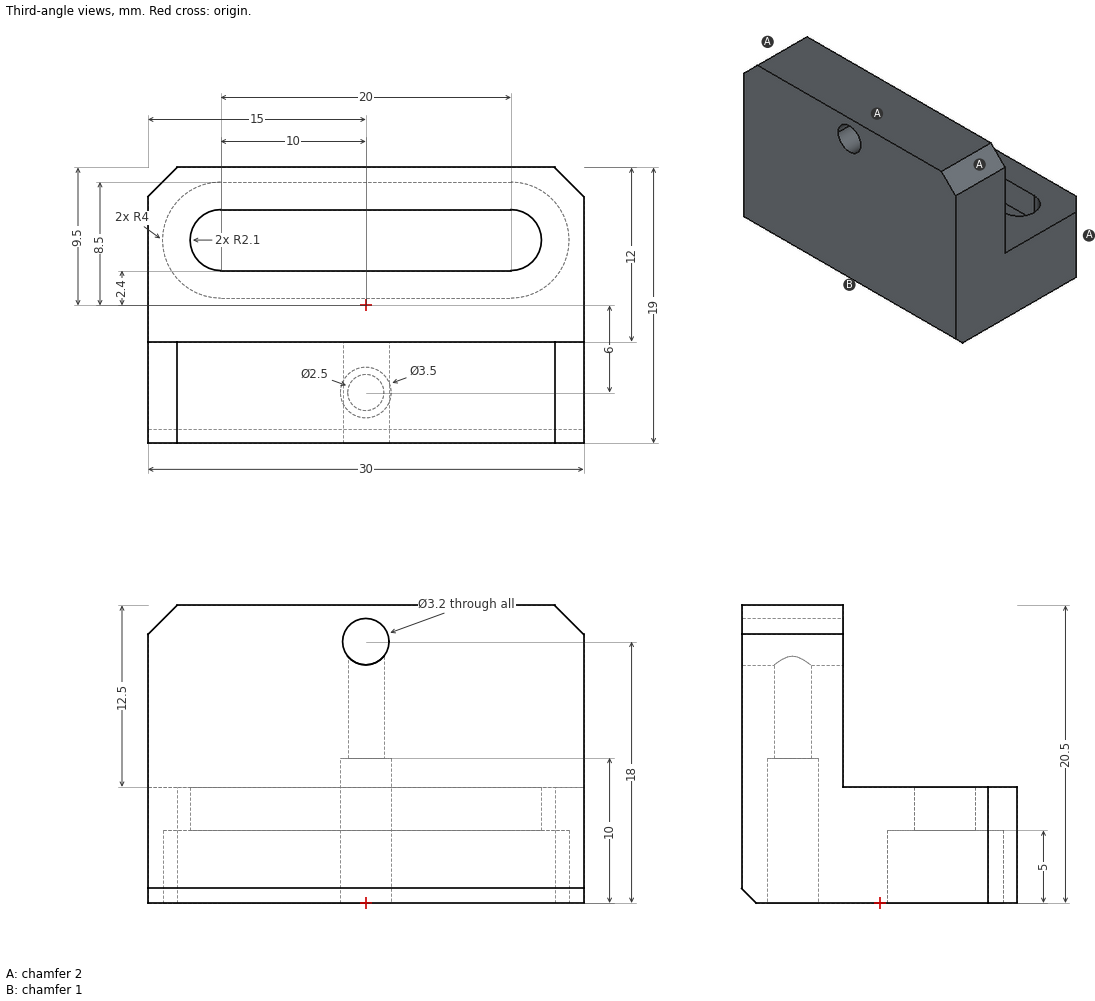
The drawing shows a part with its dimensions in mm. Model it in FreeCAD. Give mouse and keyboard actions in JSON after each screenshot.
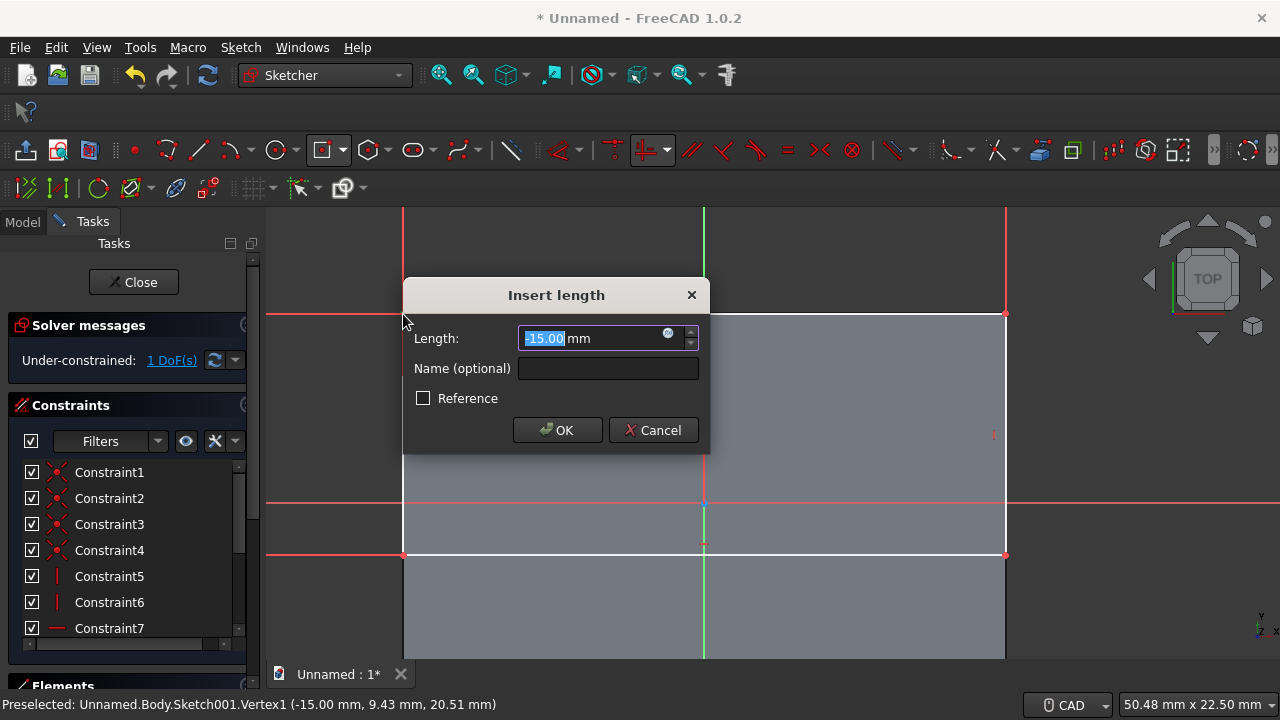
{"action": "type", "text": "-15"}
{"action": "key", "text": "Return"}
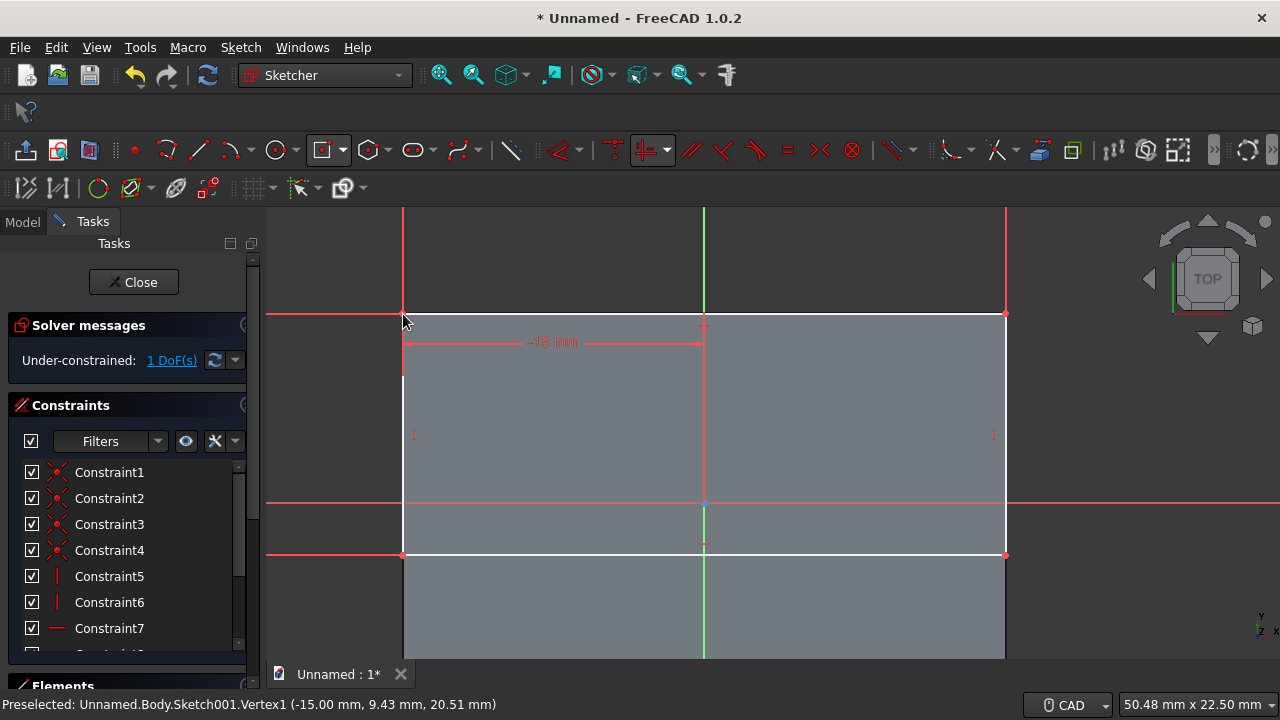
{"action": "left_click", "coordinate": [403, 314]}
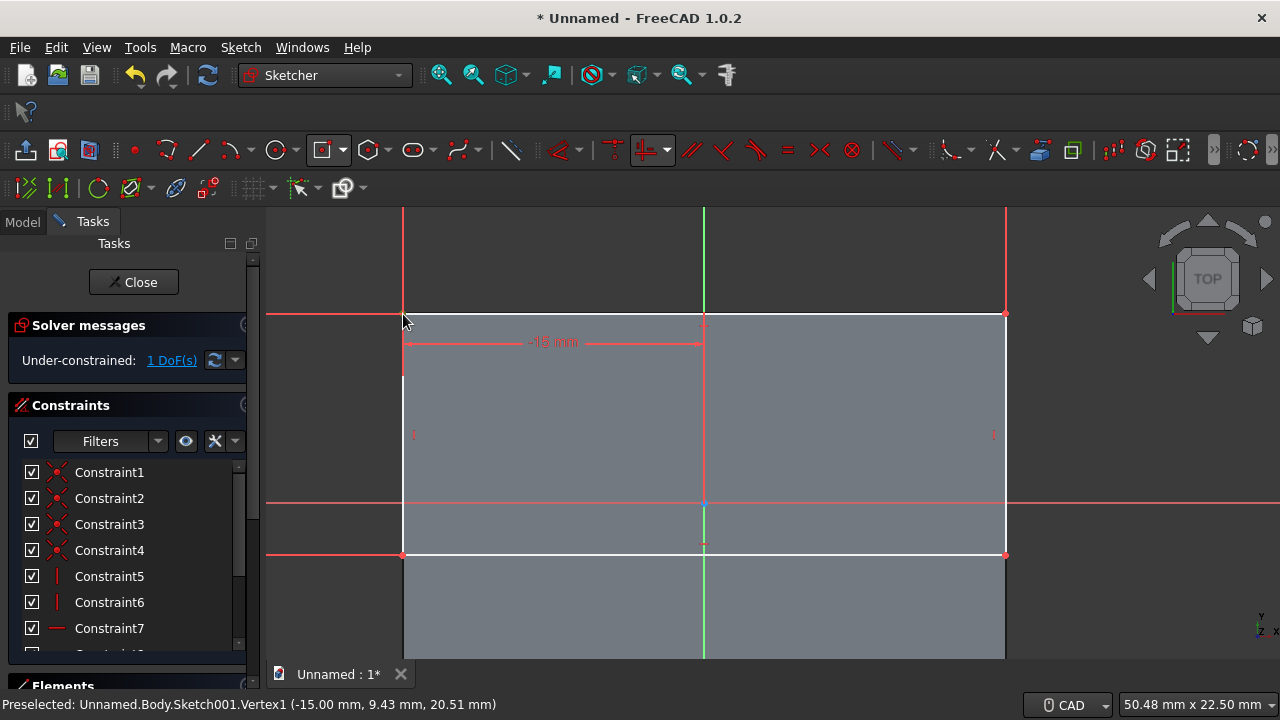
{"action": "left_click", "coordinate": [582, 150]}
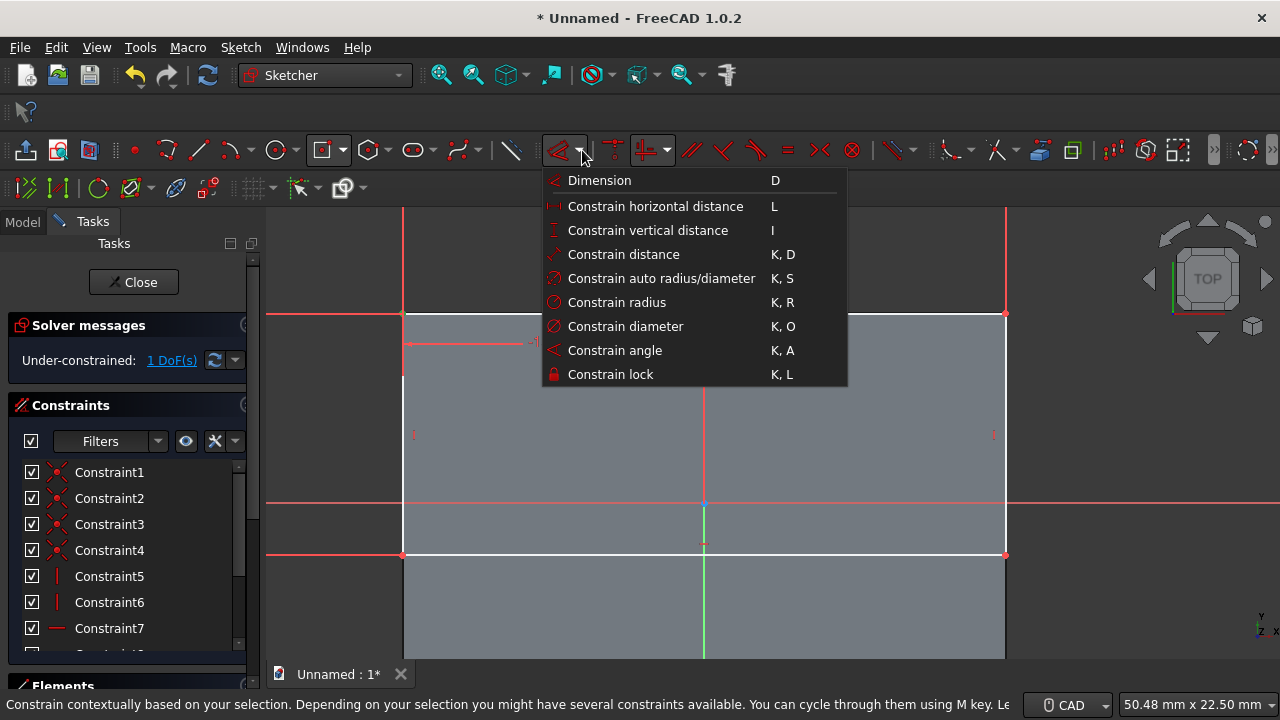
{"action": "left_click", "coordinate": [695, 230]}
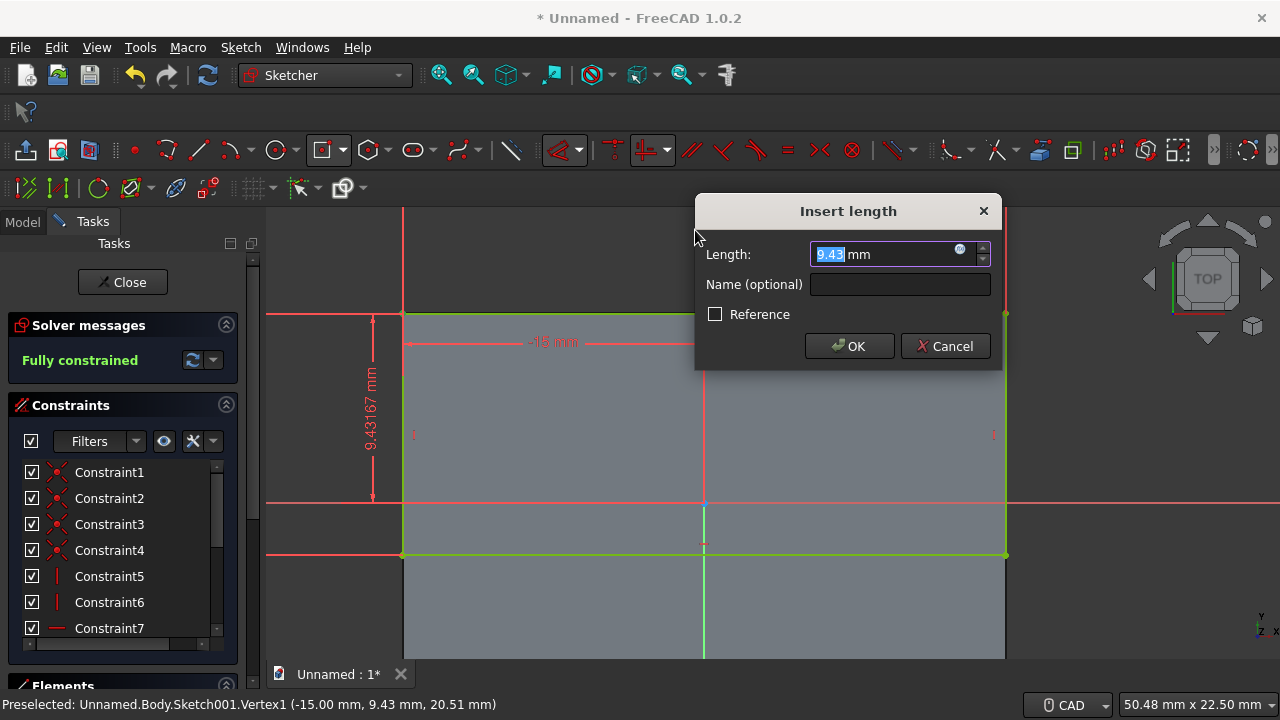
{"action": "type", "text": "9.5"}
{"action": "key", "text": "Return"}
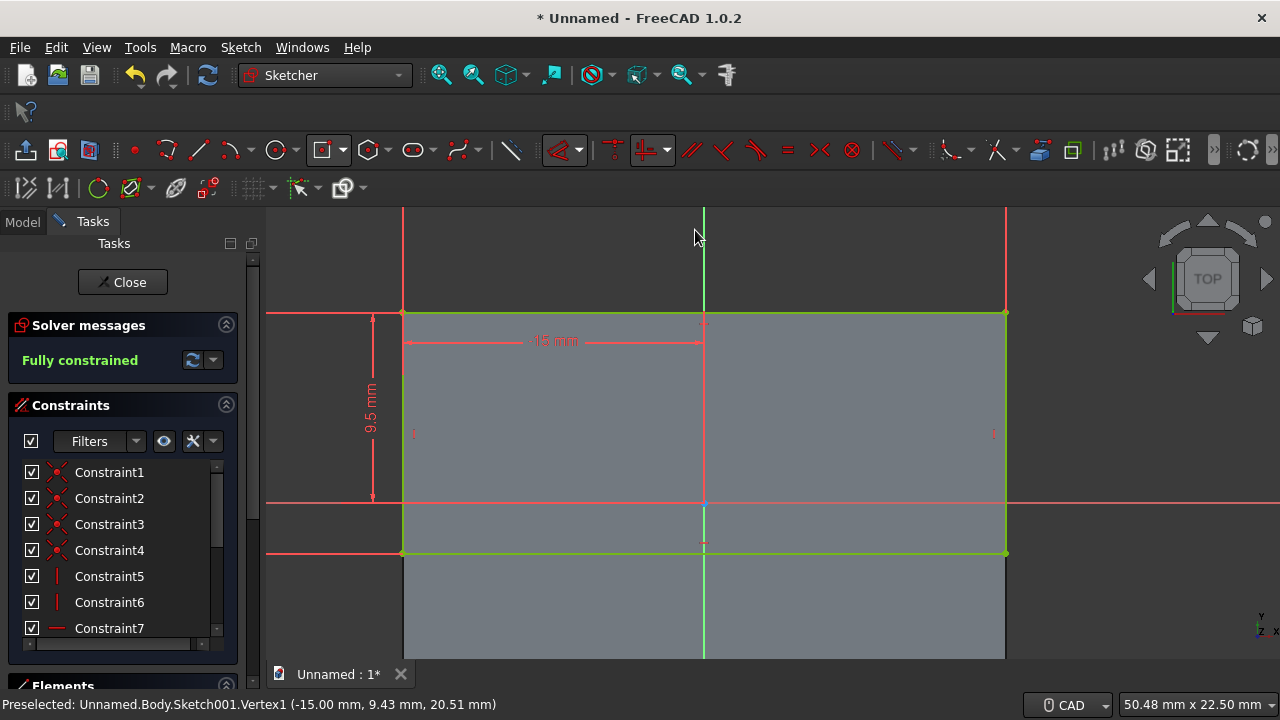
{"action": "left_click", "coordinate": [123, 282]}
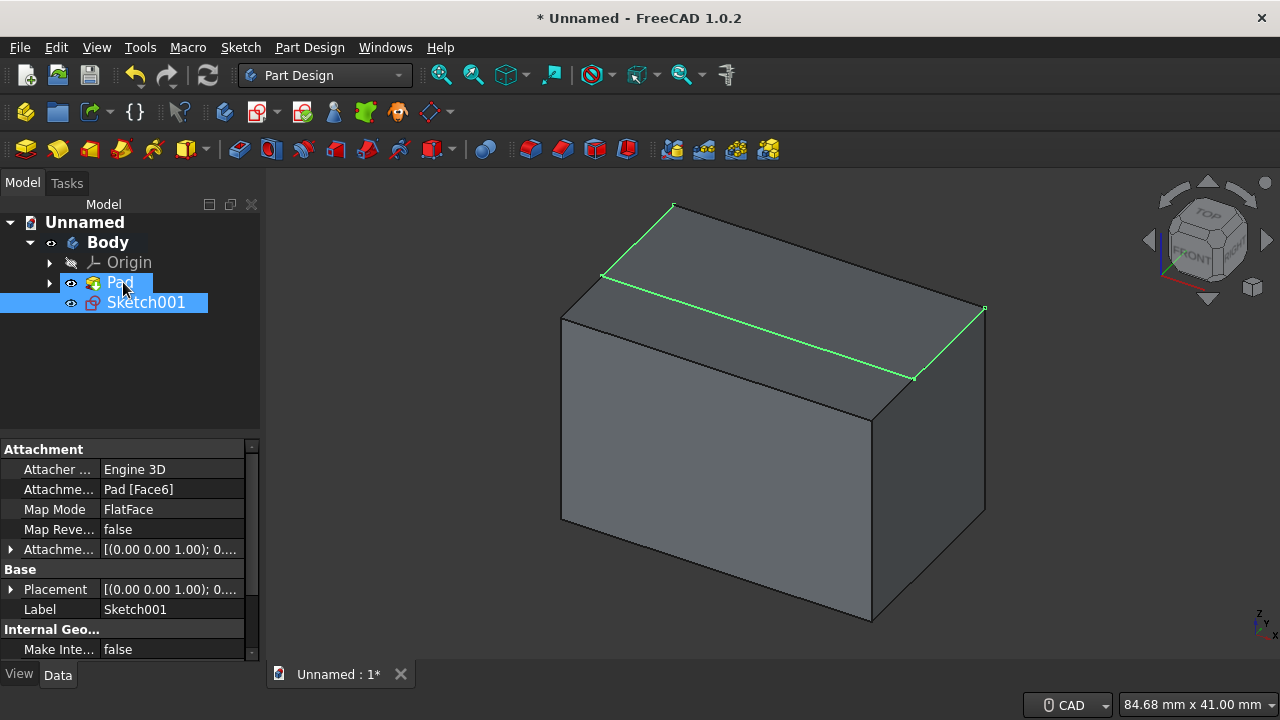
{"action": "left_click", "coordinate": [240, 150]}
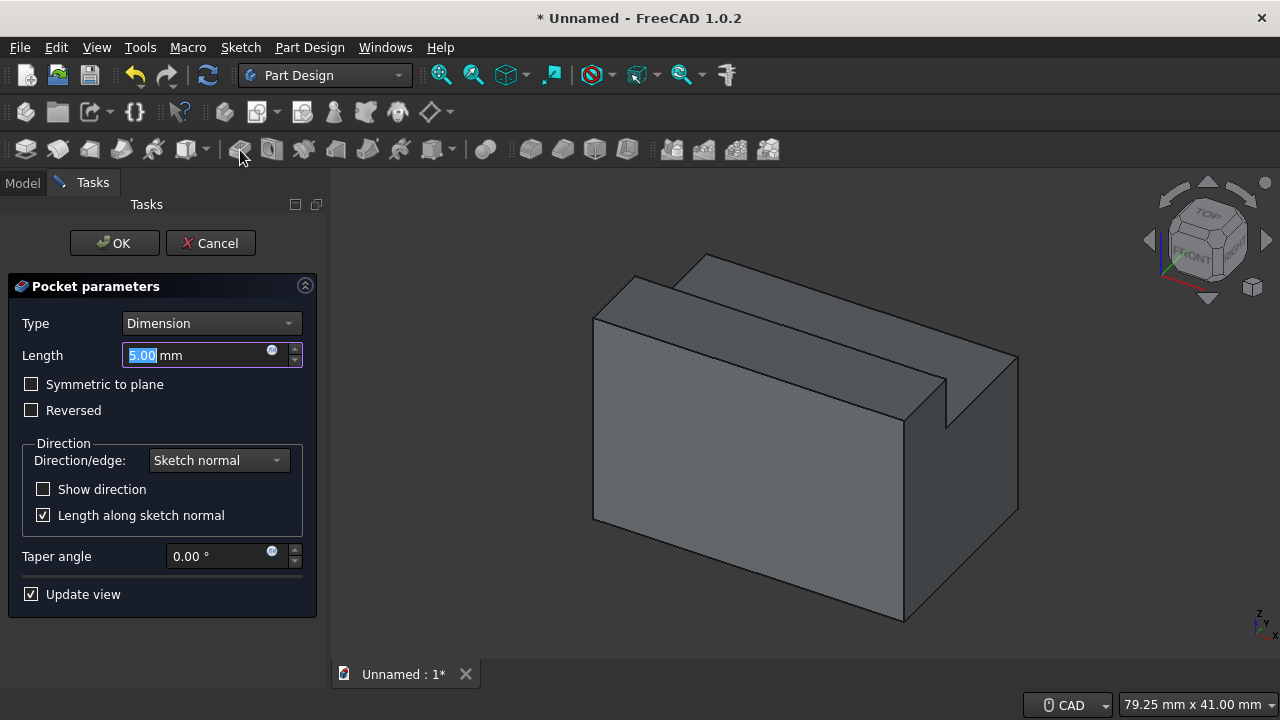
{"action": "type", "text": "12.5"}
{"action": "key", "text": "Tab"}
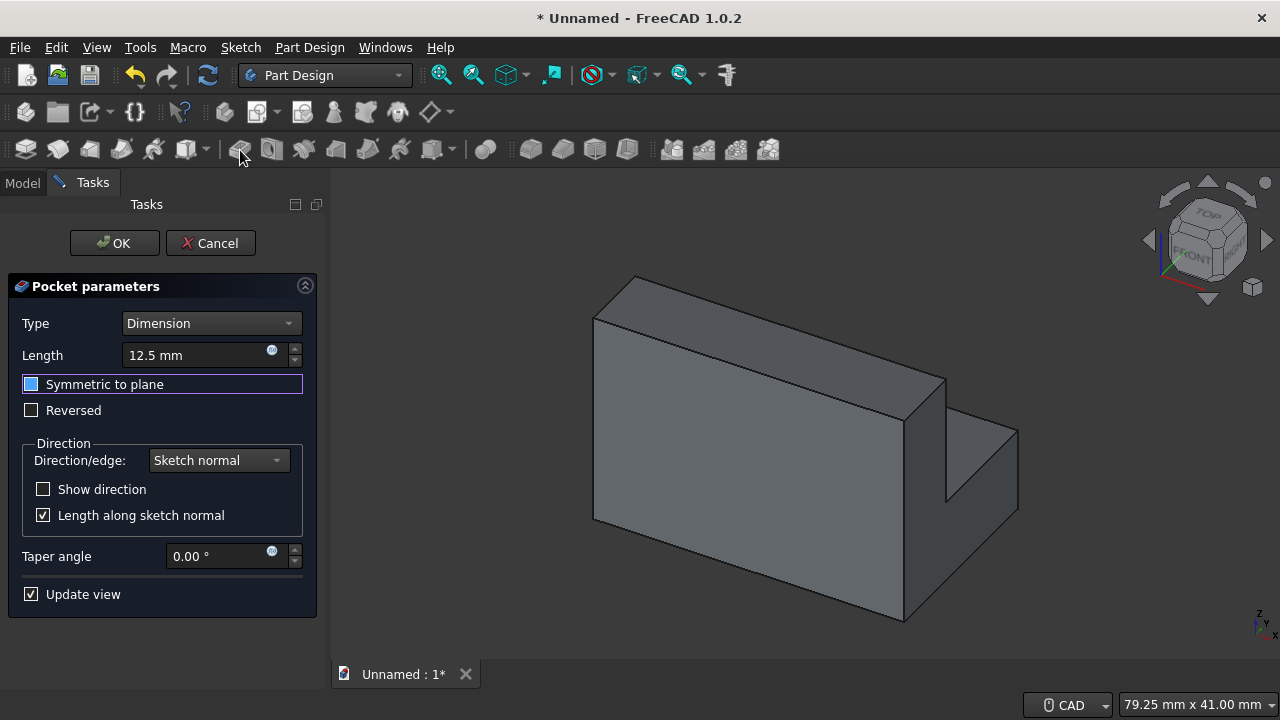
{"action": "left_click", "coordinate": [115, 243]}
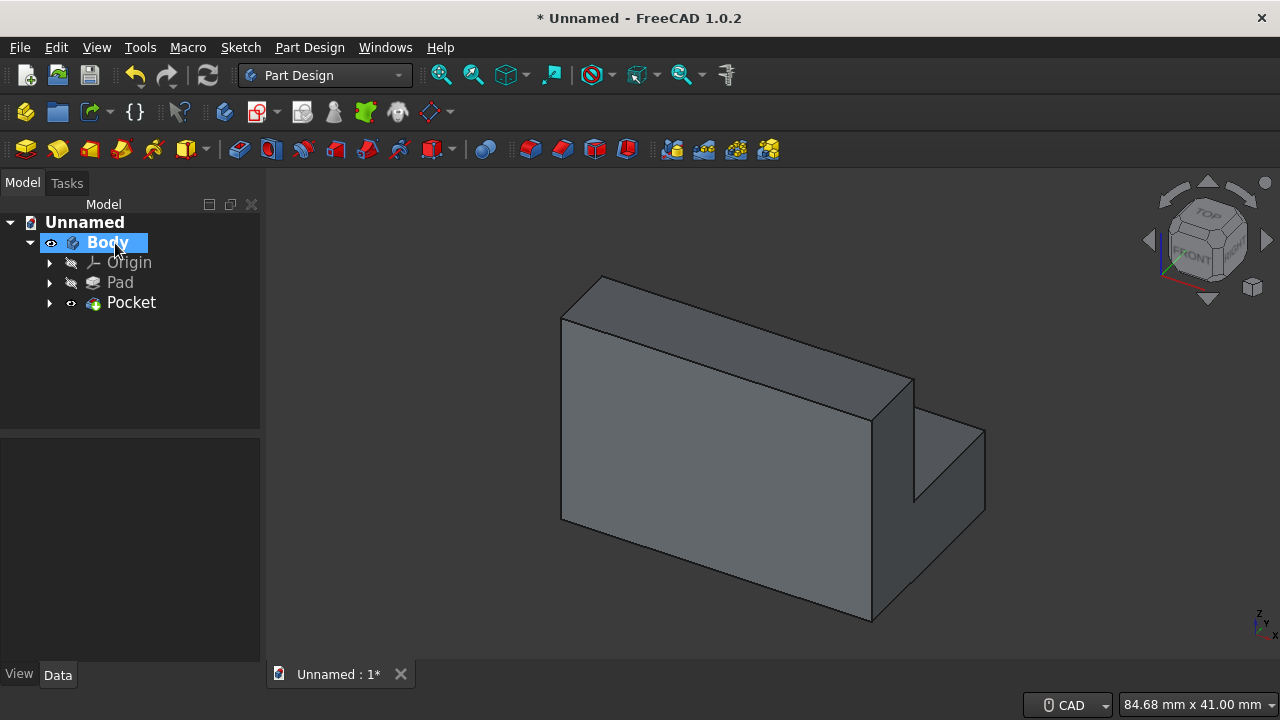
{"action": "key", "text": "5"}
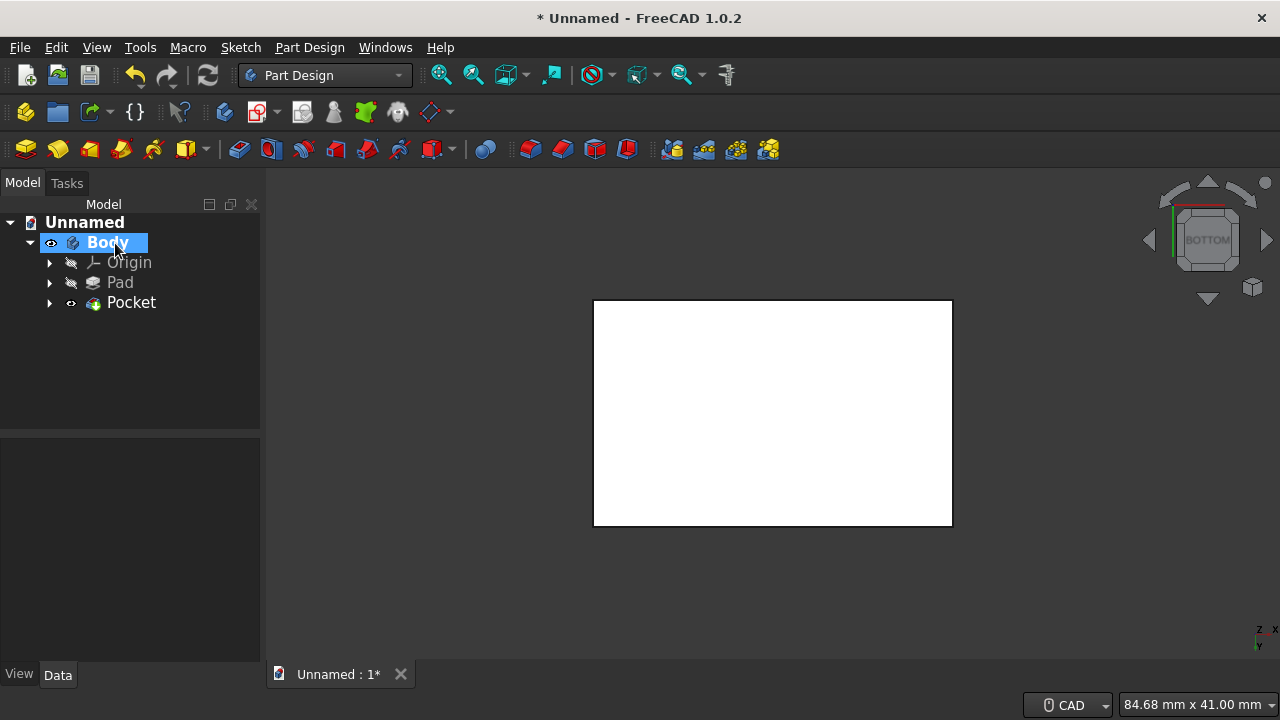
{"action": "left_click", "coordinate": [824, 412]}